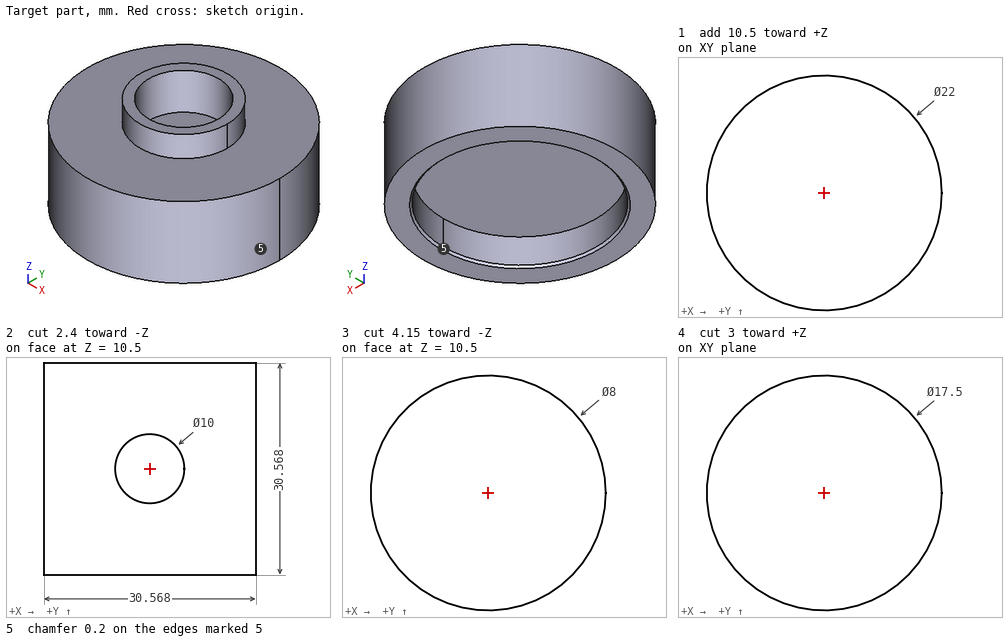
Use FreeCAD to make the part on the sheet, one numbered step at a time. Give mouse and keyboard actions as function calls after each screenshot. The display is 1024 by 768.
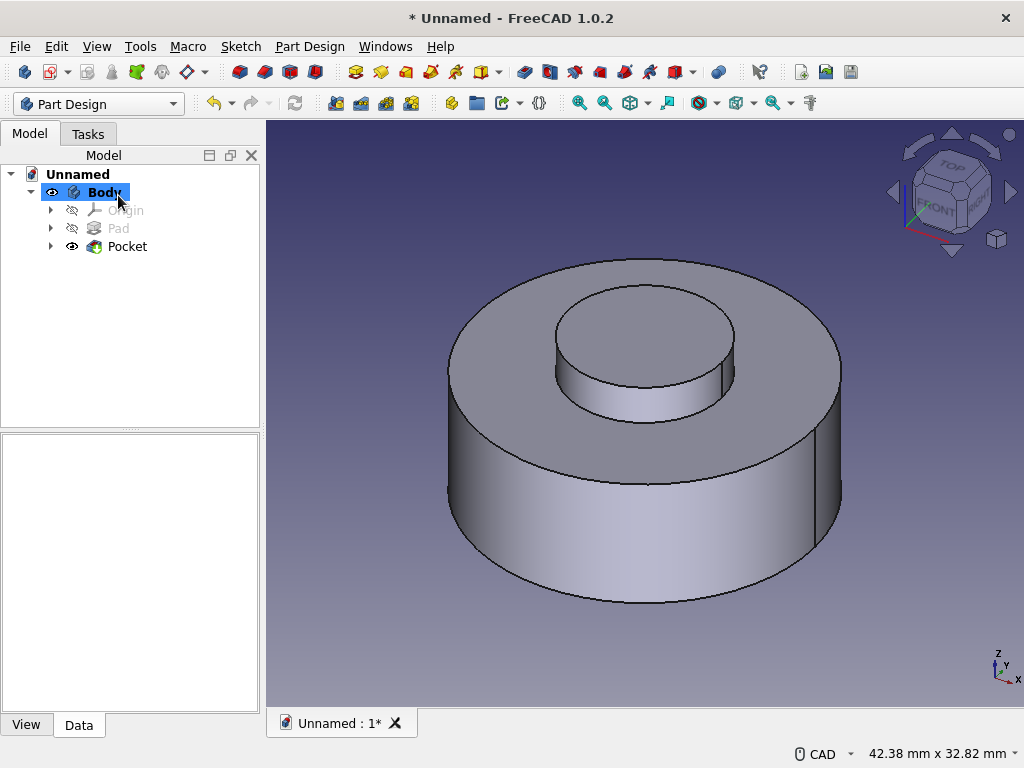
click(645, 336)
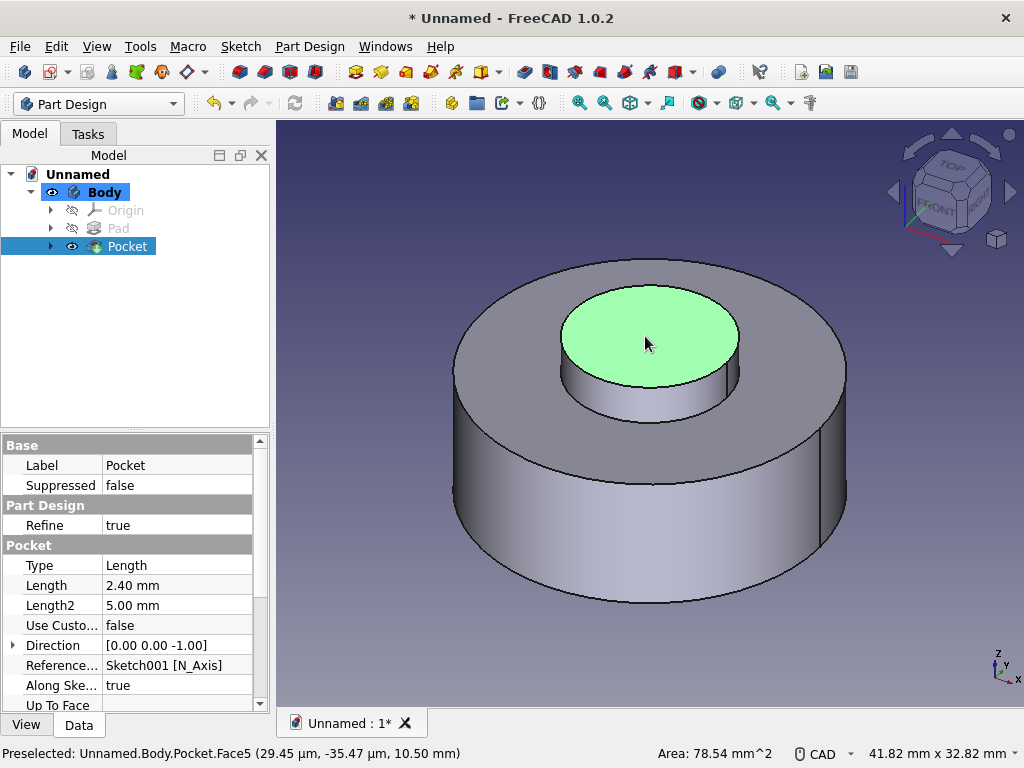
click(50, 72)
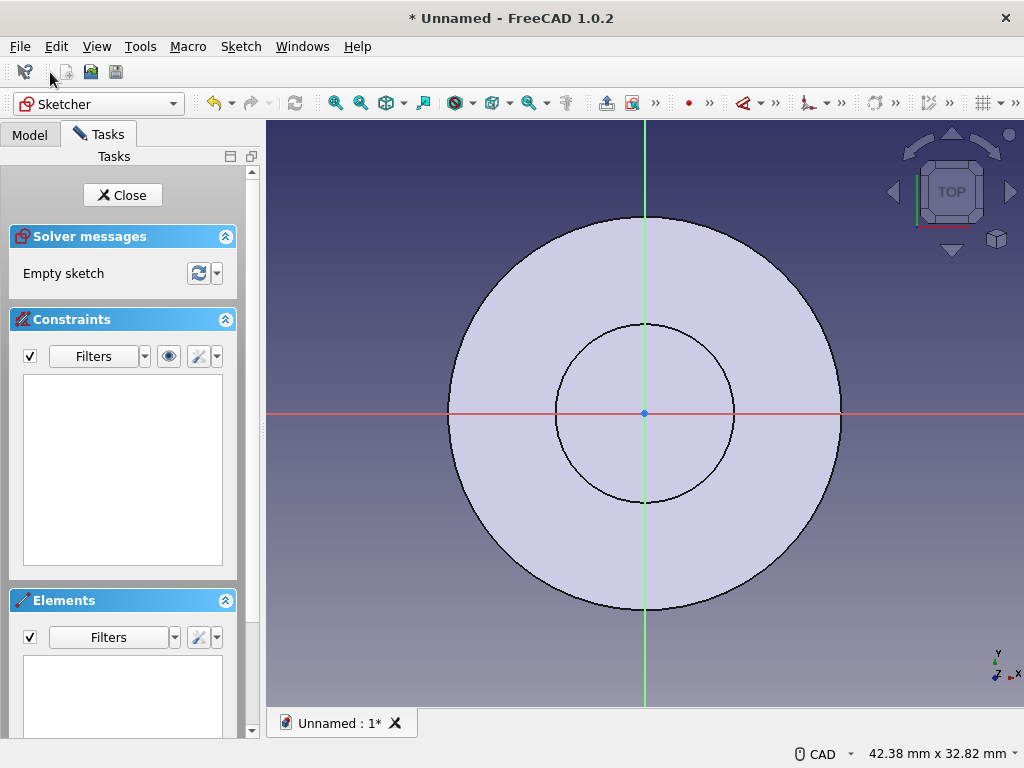
scroll(685, 414, up, 5)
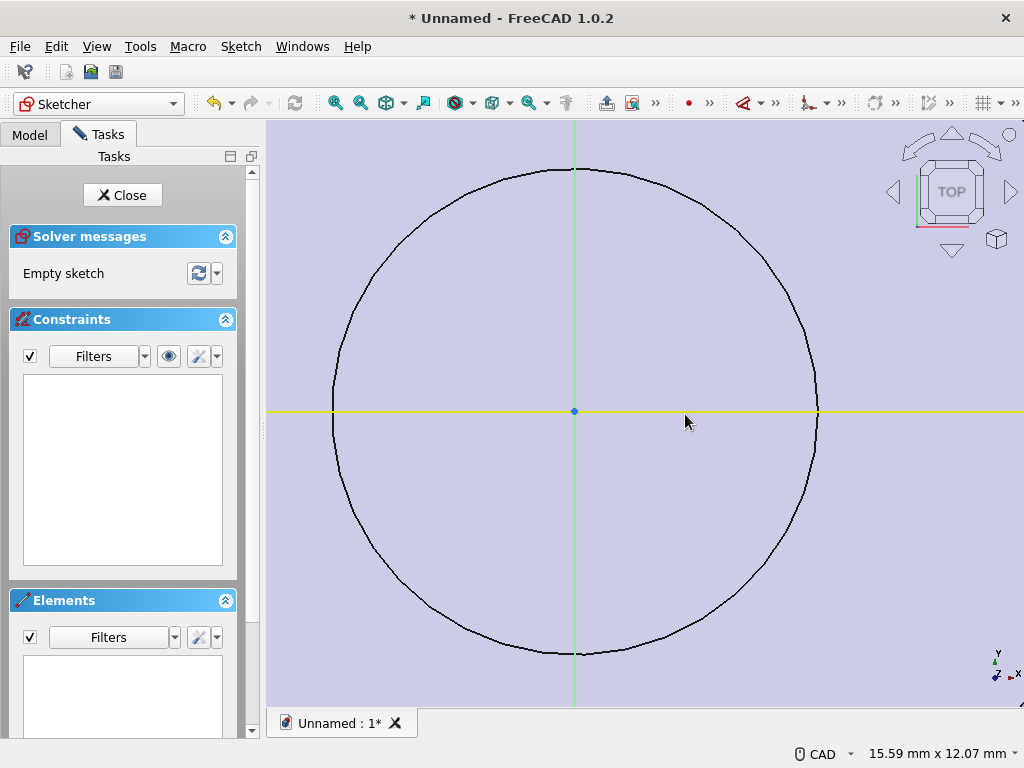
key(g)
key(c)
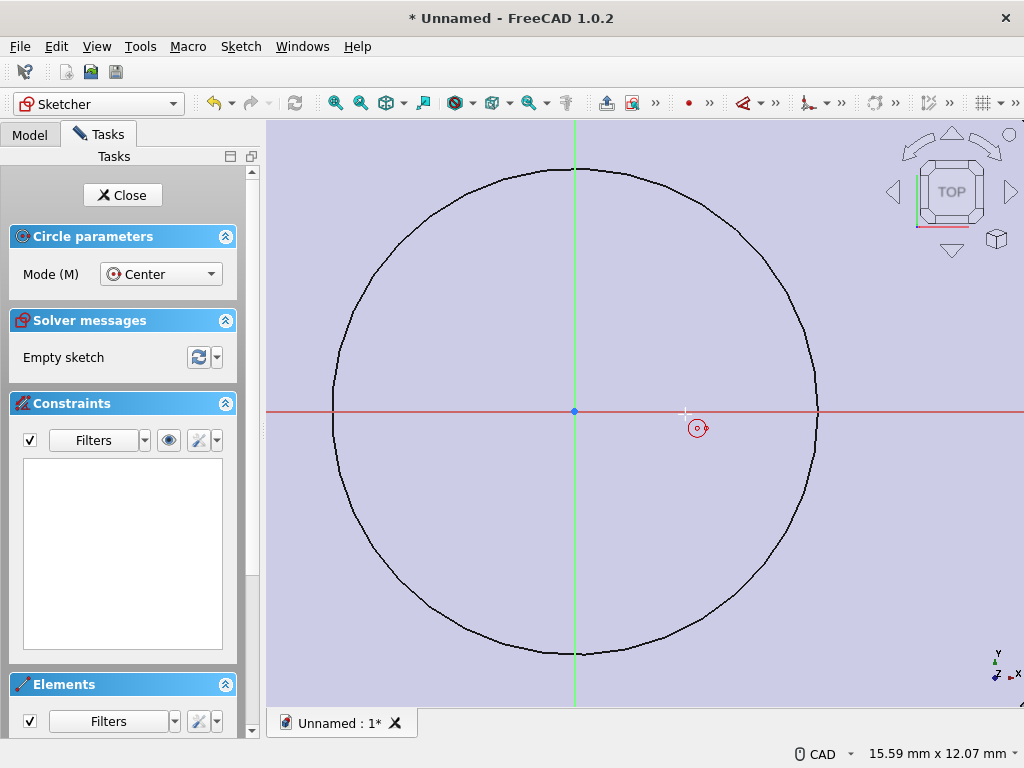
click(575, 412)
move(712, 274)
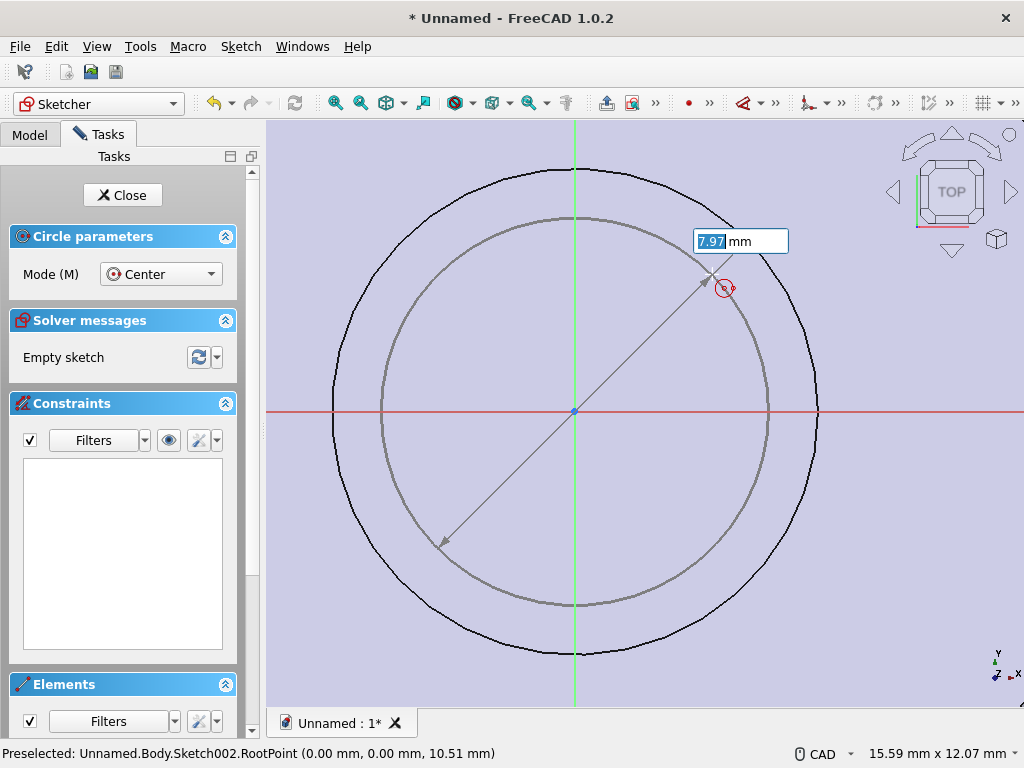
text(8)
key(Return)
key(Escape)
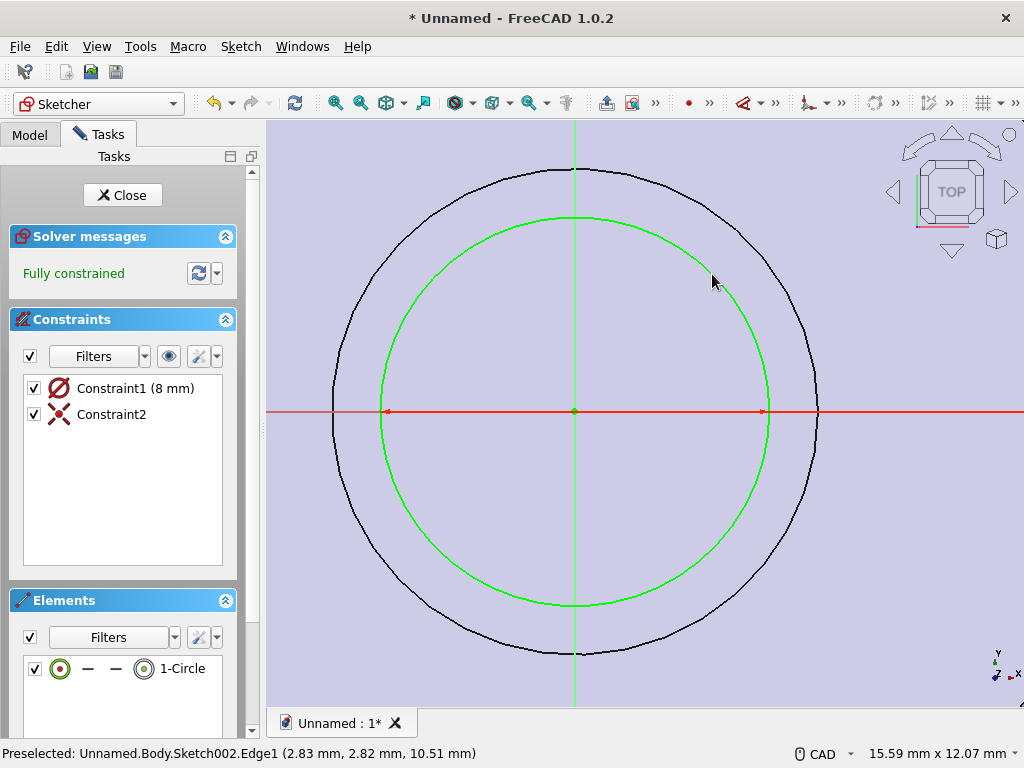
click(123, 195)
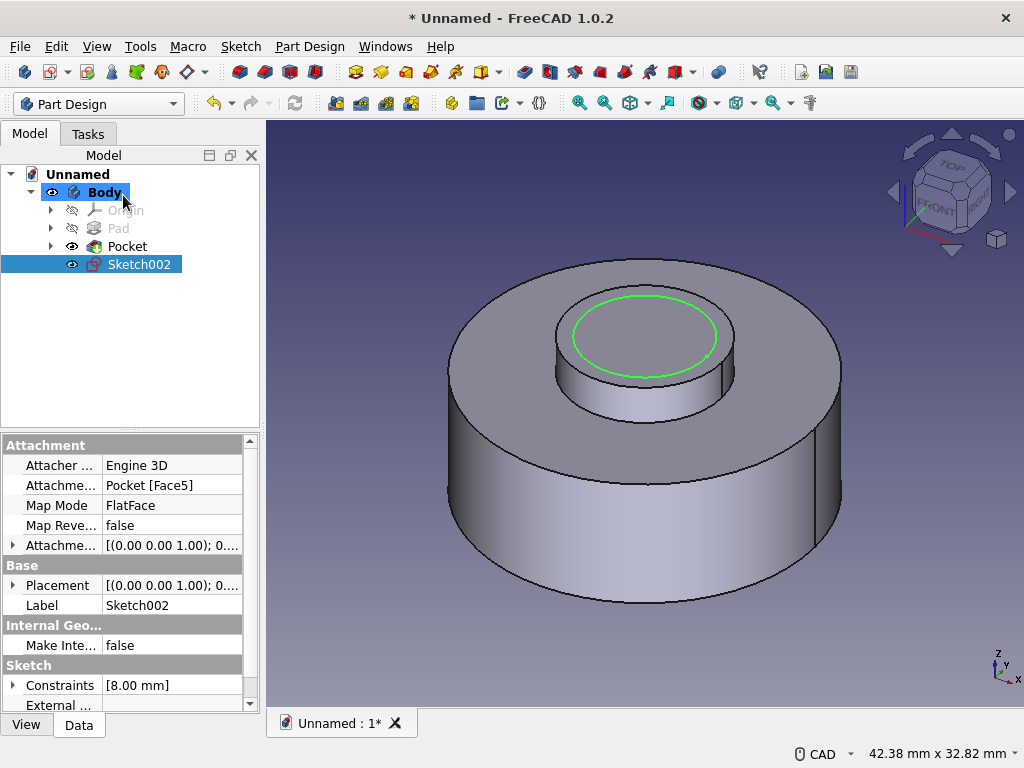
click(525, 72)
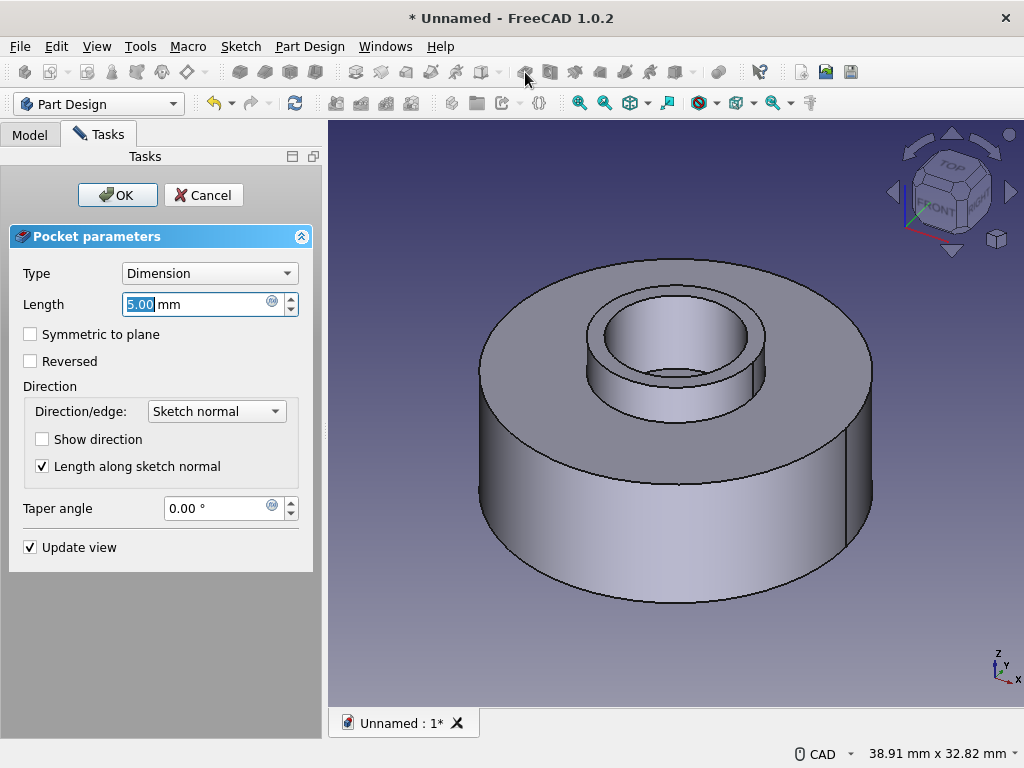
text(4.15)
key(Tab)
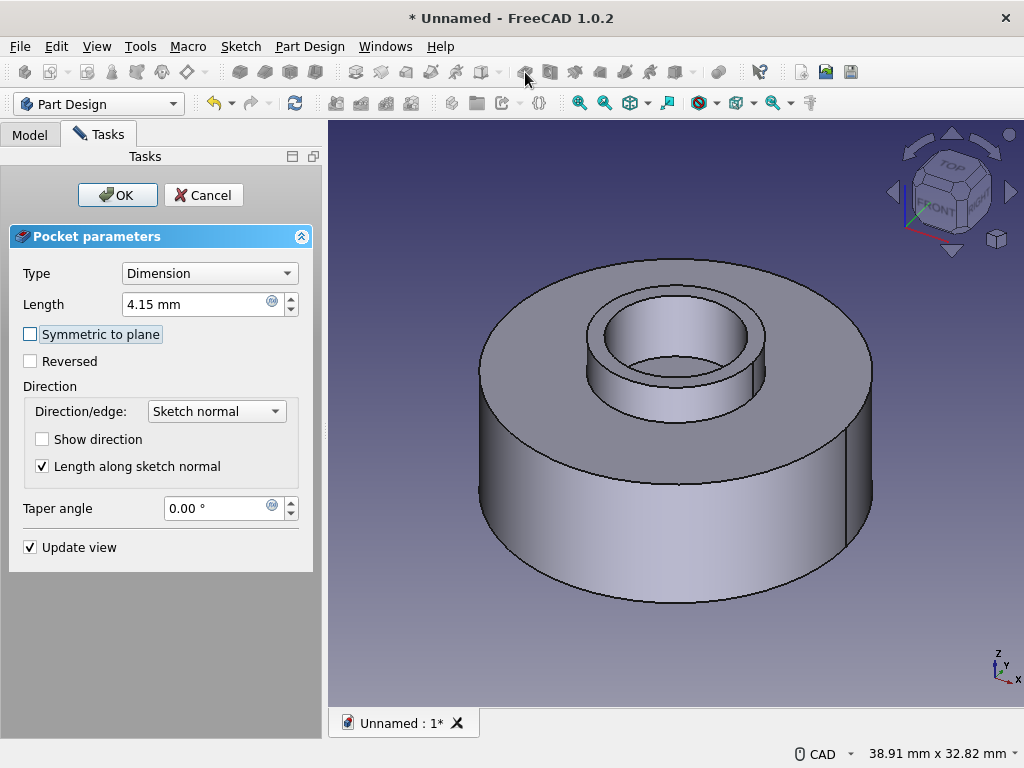
click(118, 195)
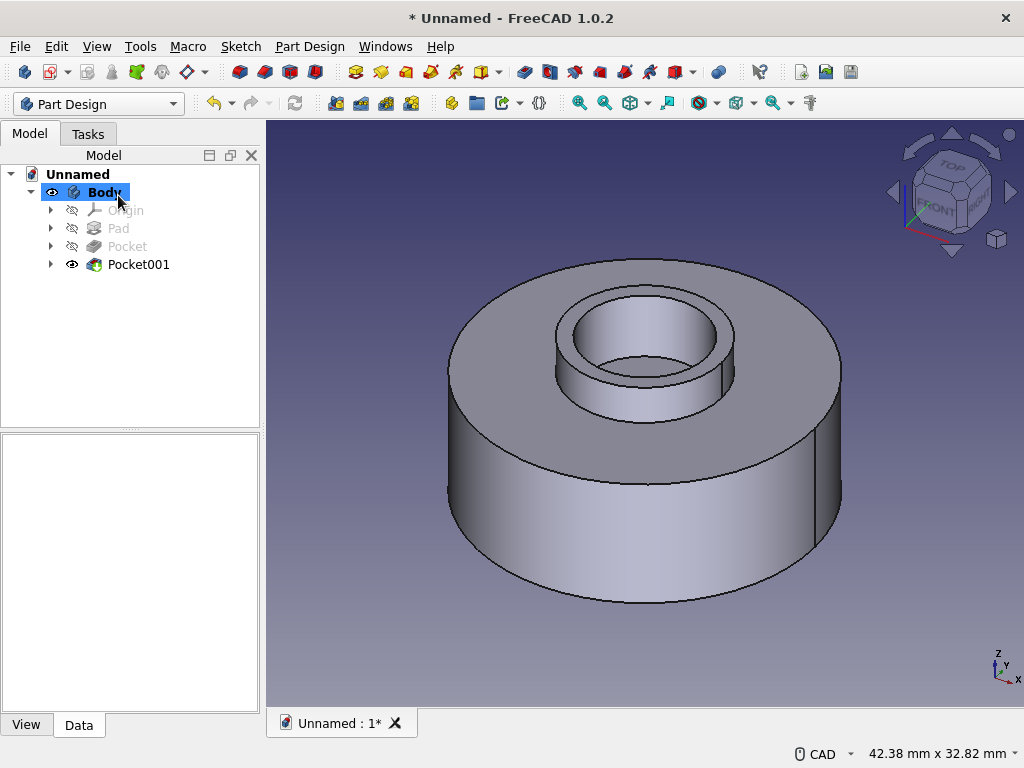
click(50, 72)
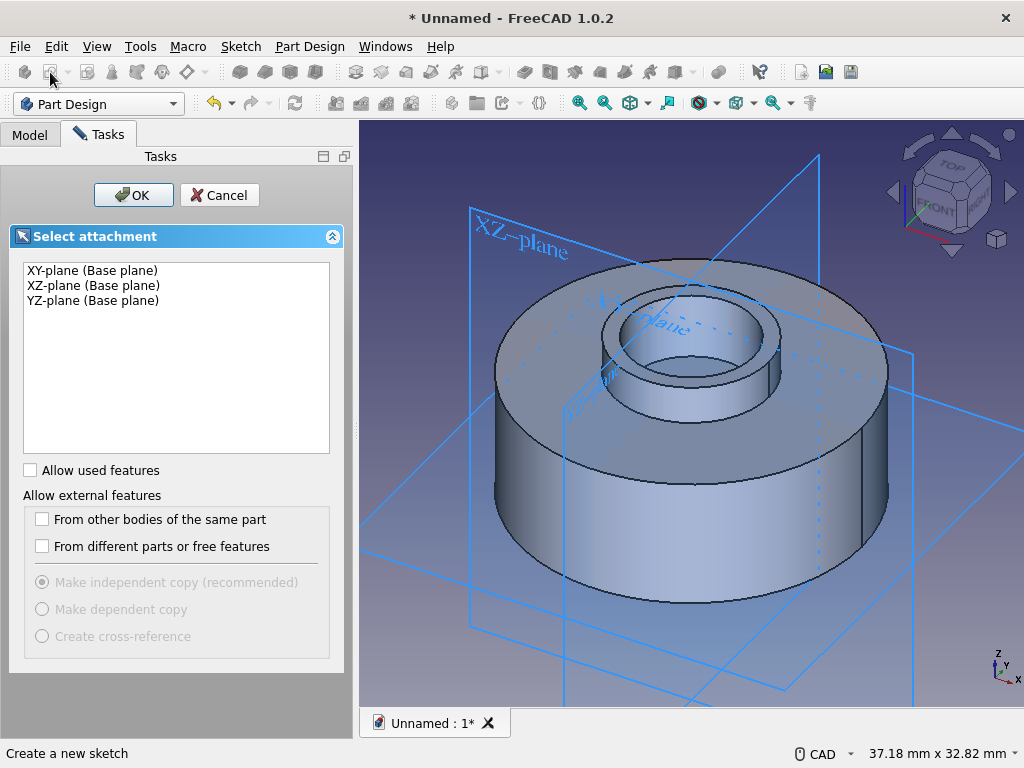
click(84, 270)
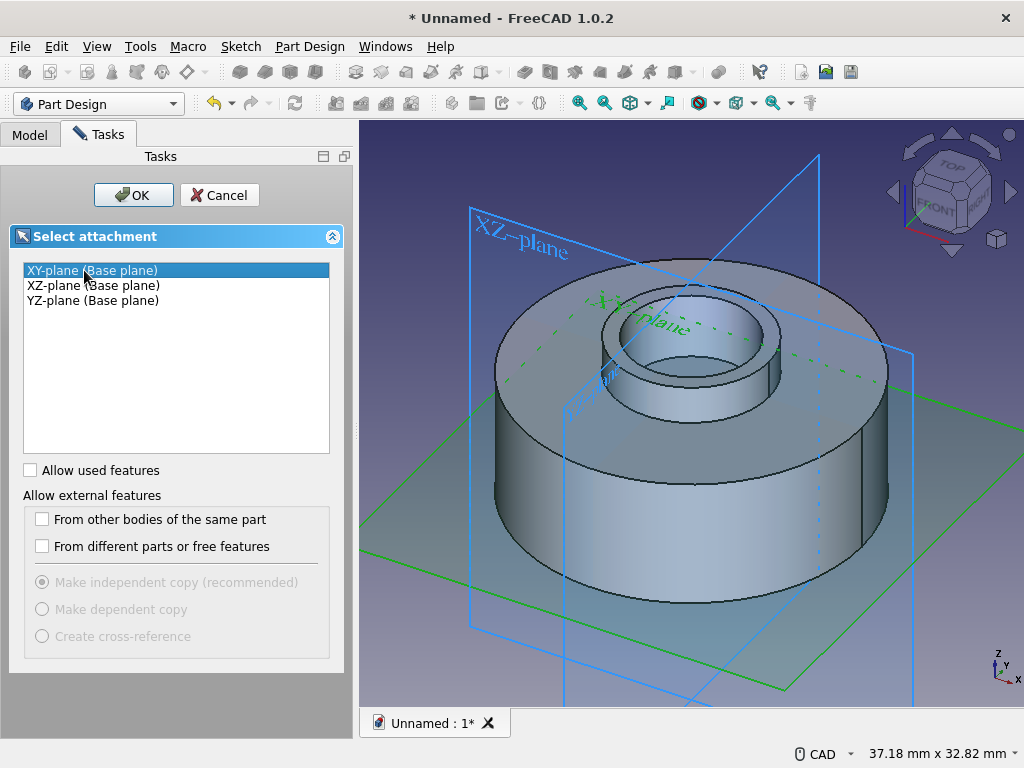
click(134, 195)